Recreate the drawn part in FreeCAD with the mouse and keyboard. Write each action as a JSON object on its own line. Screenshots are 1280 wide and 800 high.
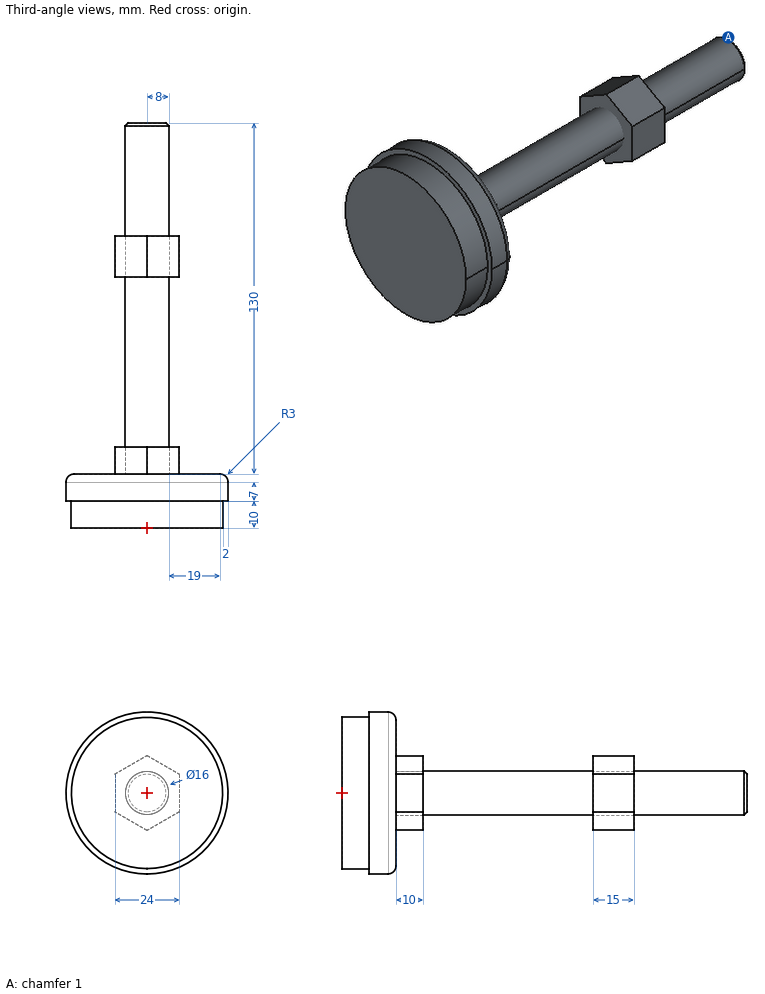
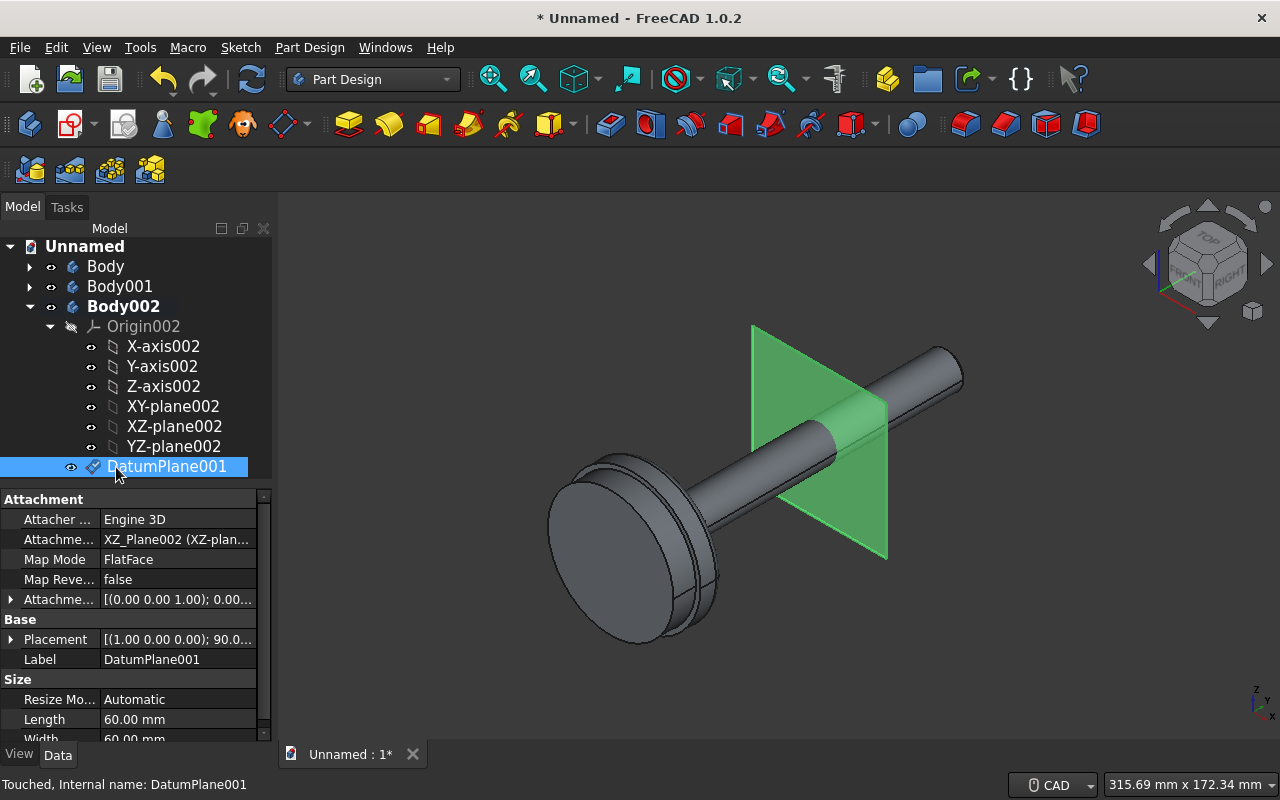
{"action": "left_click", "coordinate": [70, 124]}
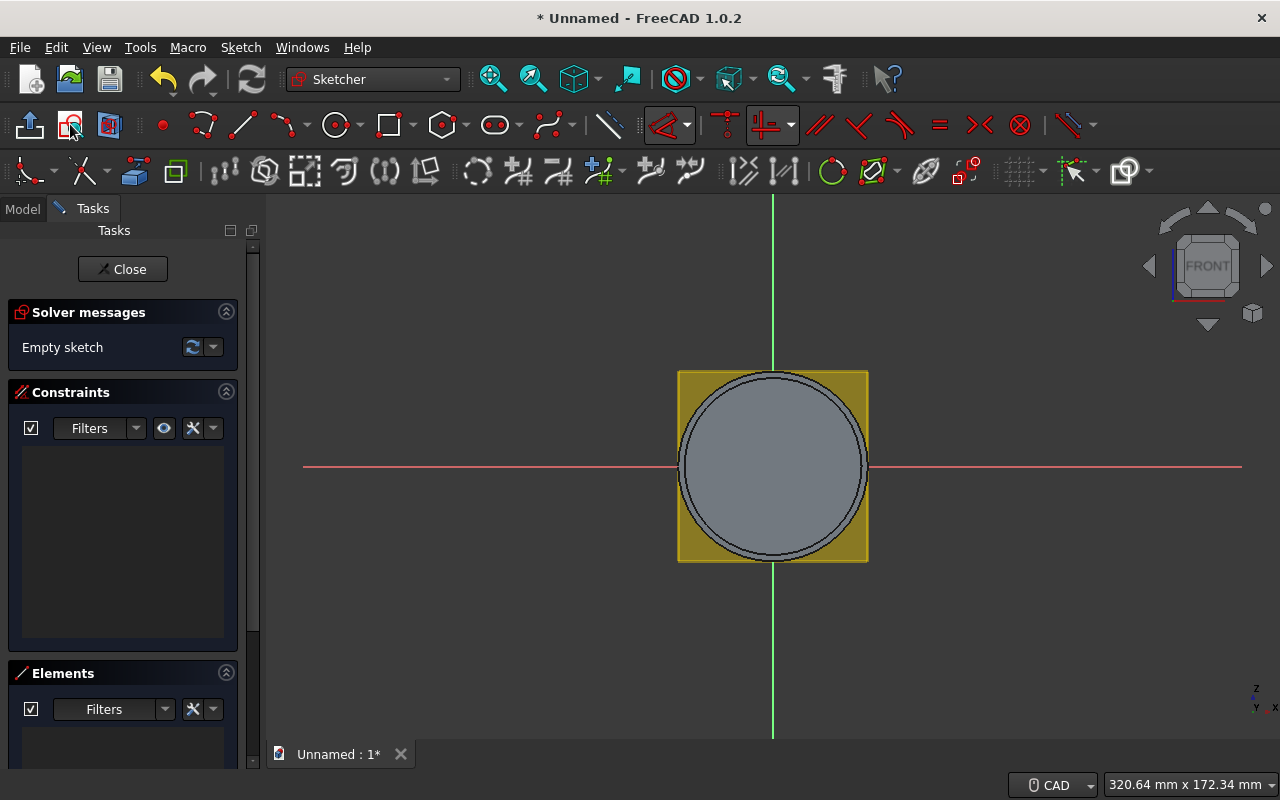
{"action": "scroll", "coordinate": [795, 467], "scroll_direction": "up", "scroll_amount": 7}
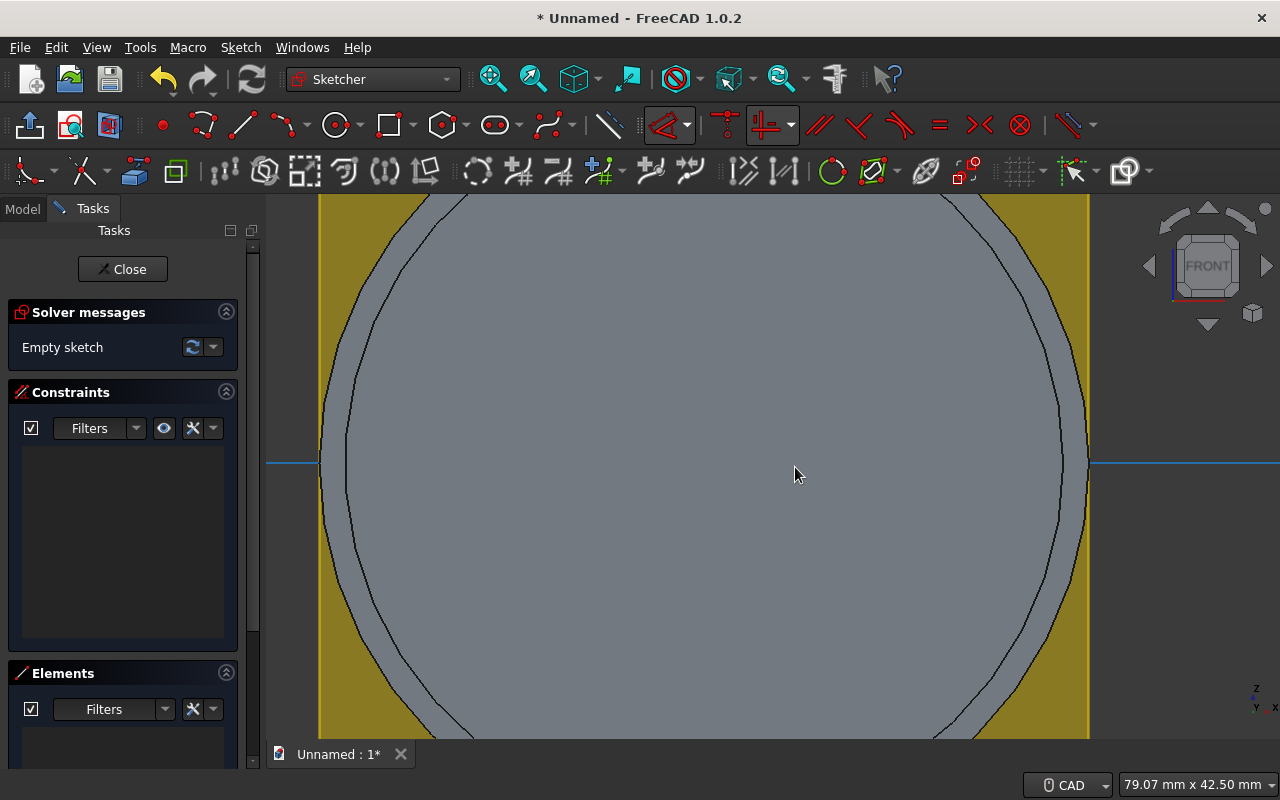
{"action": "left_click", "coordinate": [442, 126]}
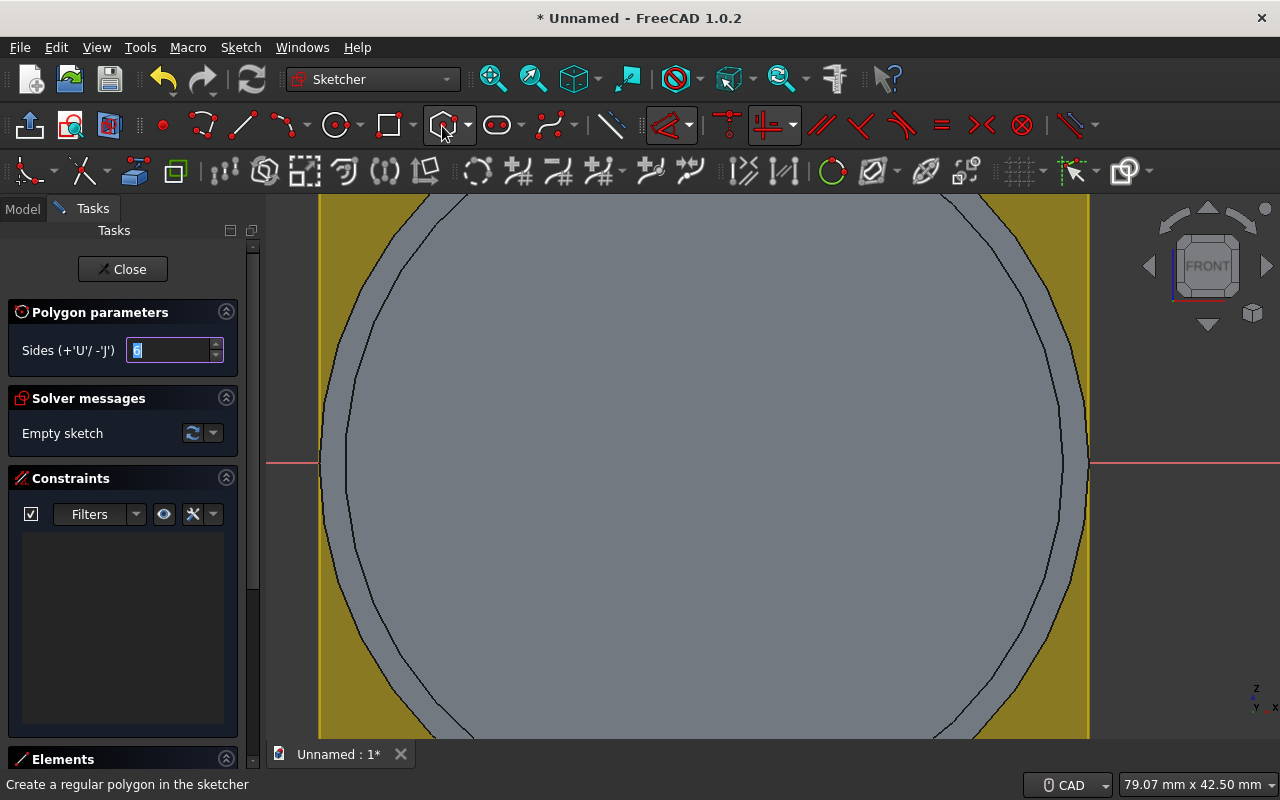
{"action": "left_click", "coordinate": [704, 463]}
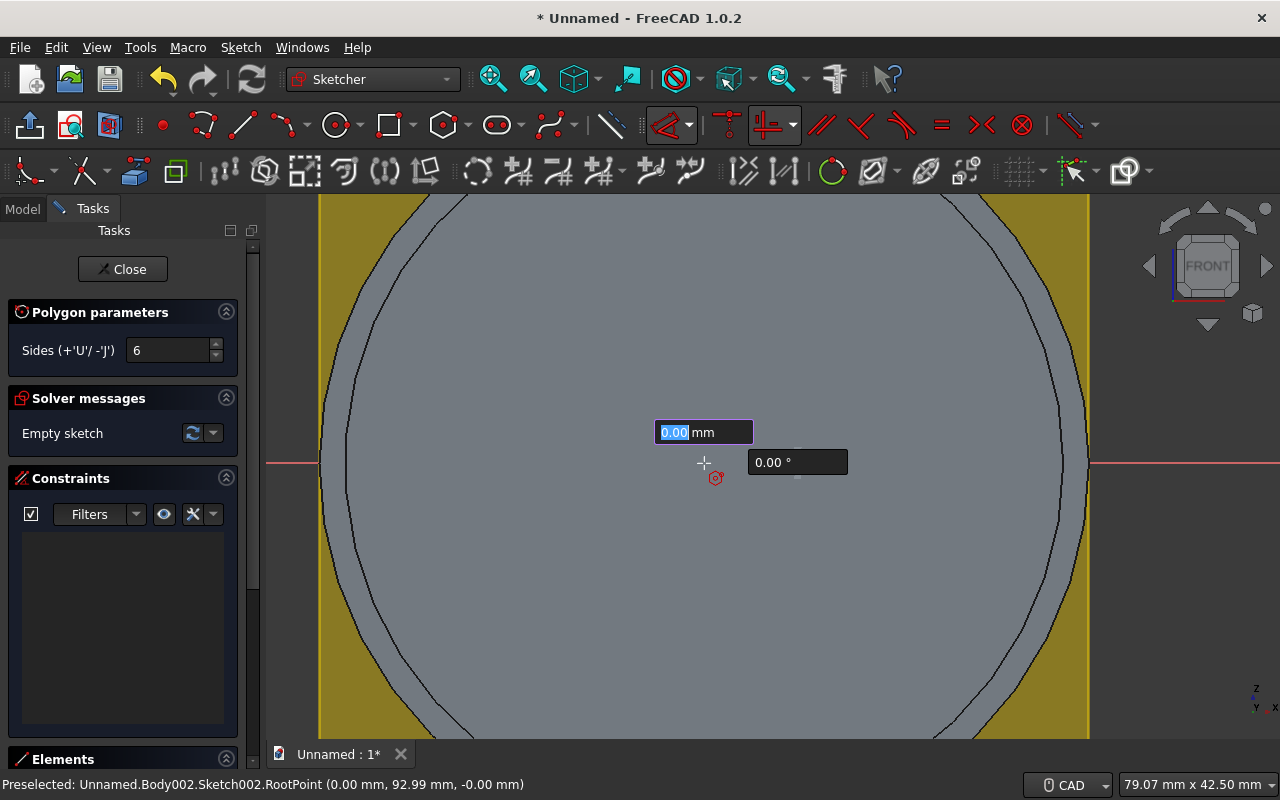
{"action": "left_click", "coordinate": [704, 641]}
{"action": "key", "text": "Escape"}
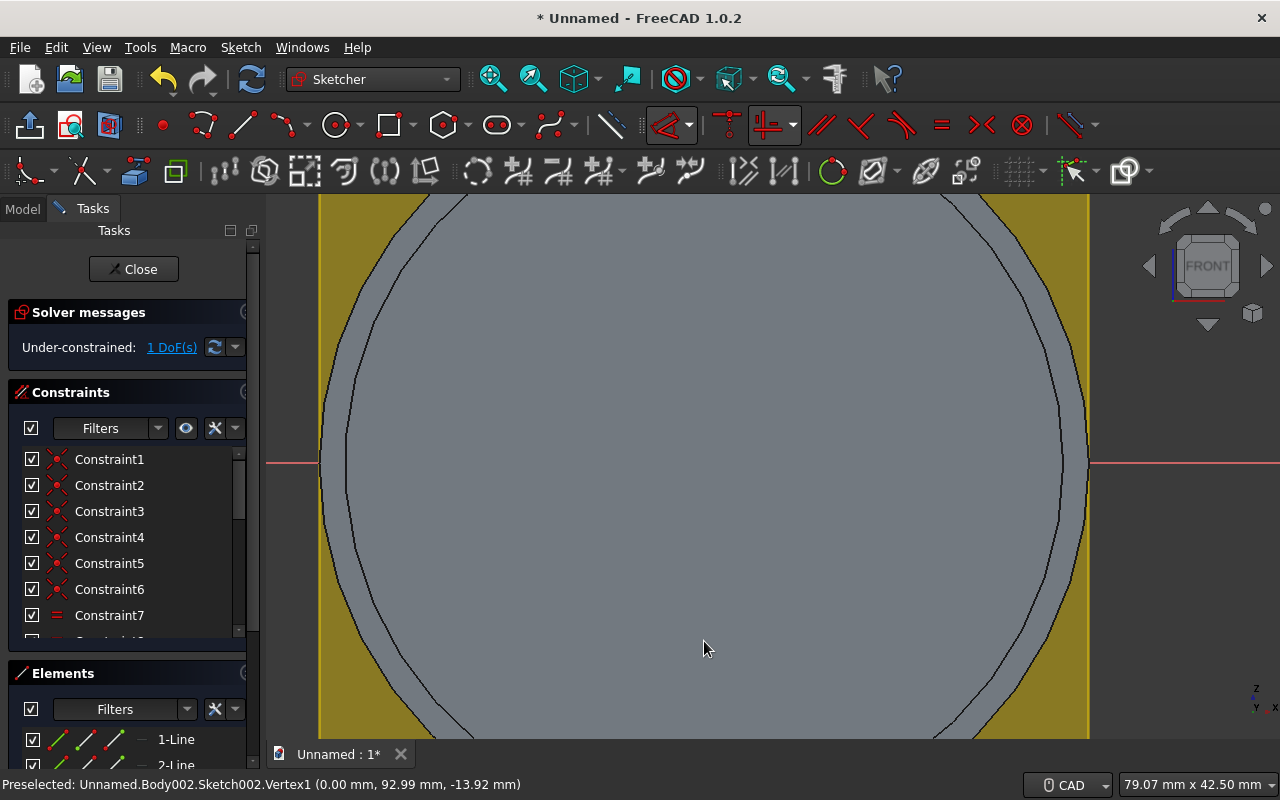
{"action": "left_click", "coordinate": [550, 374]}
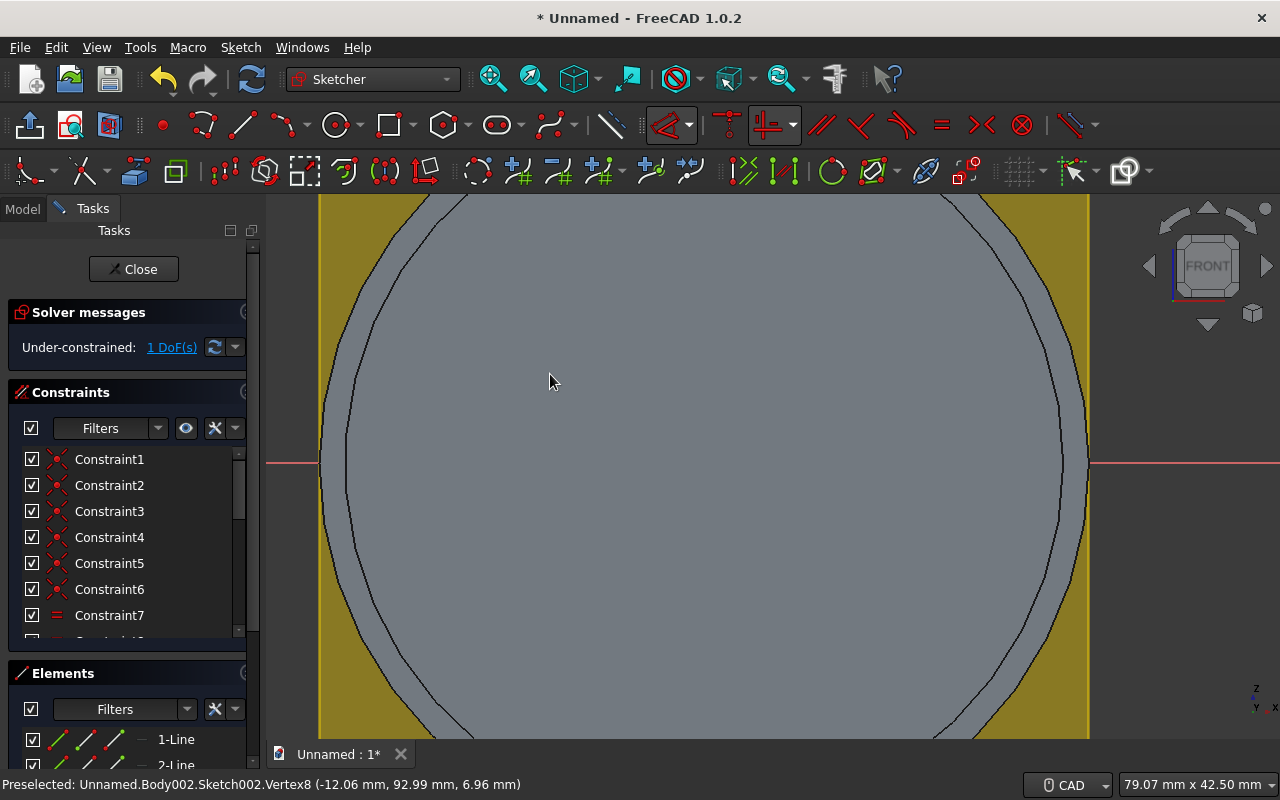
{"action": "left_click", "coordinate": [859, 553]}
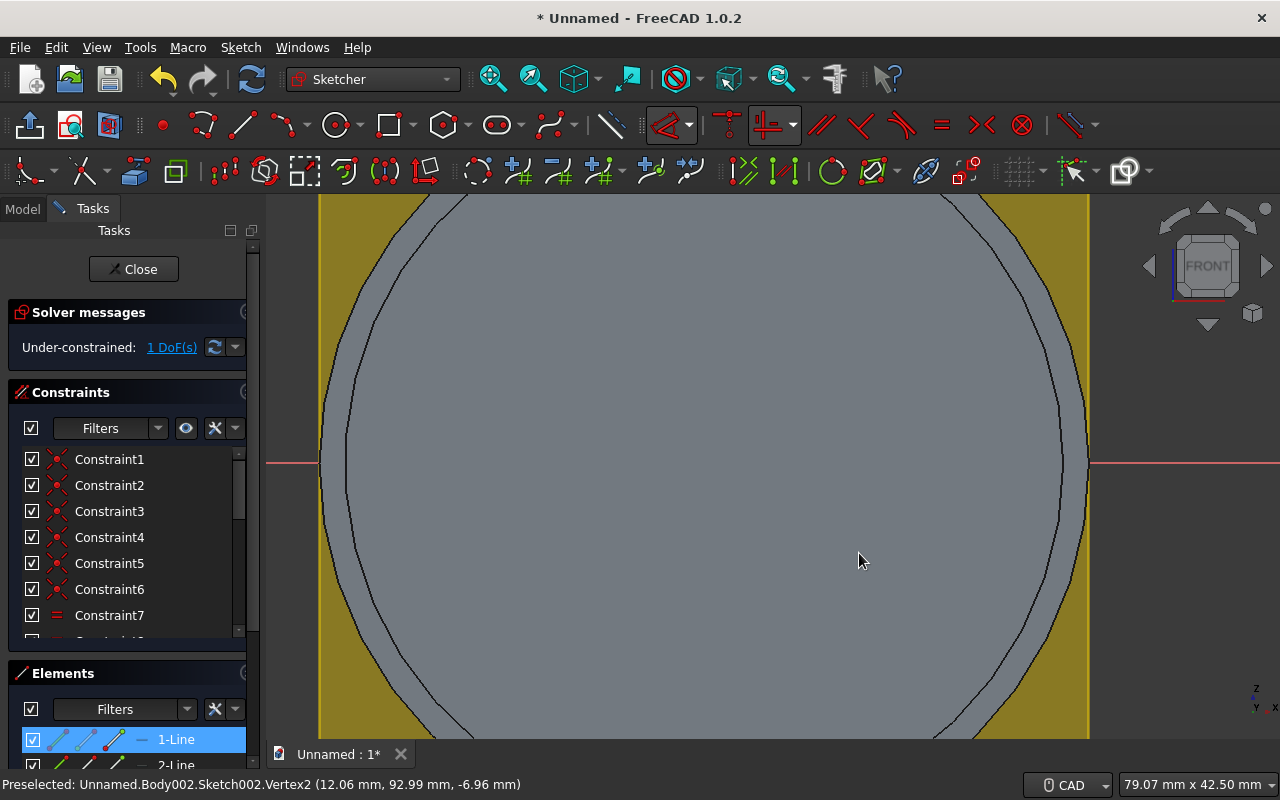
{"action": "key", "text": "l"}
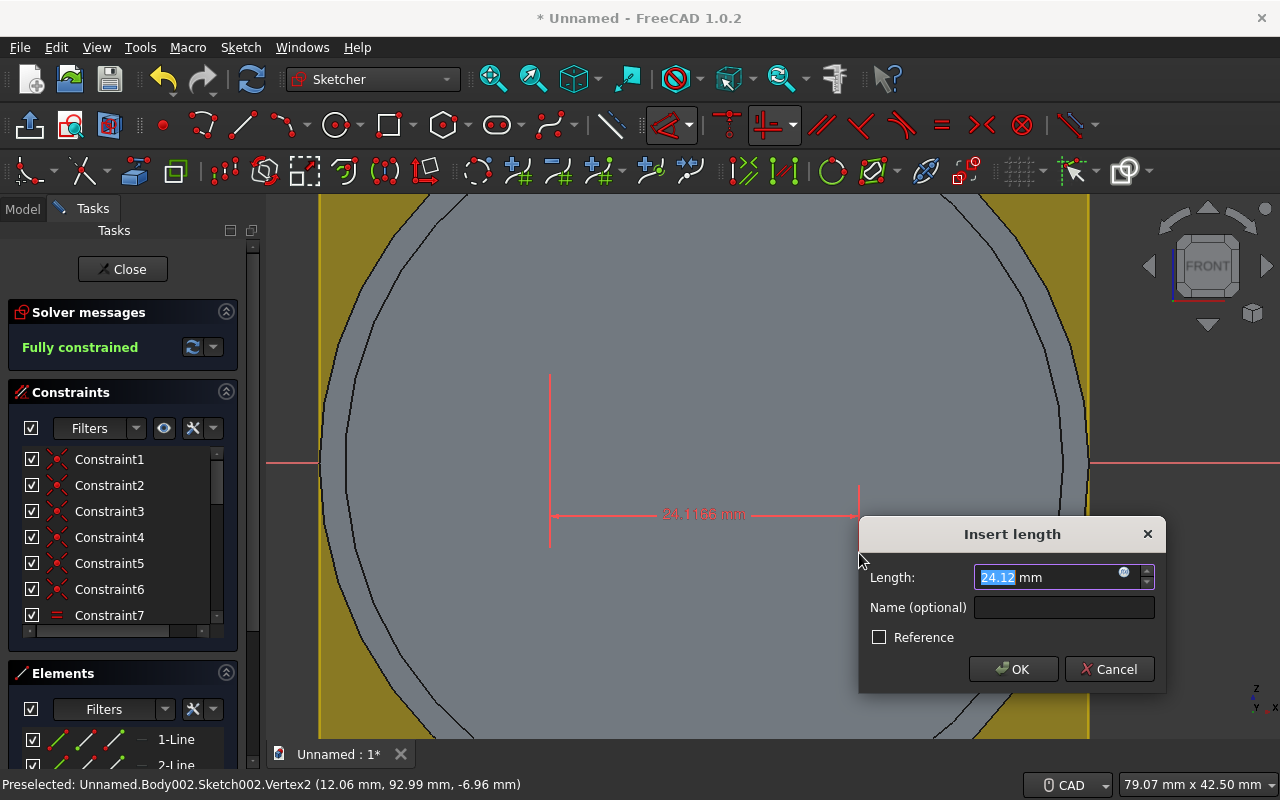
{"action": "type", "text": "24"}
{"action": "key", "text": "Return"}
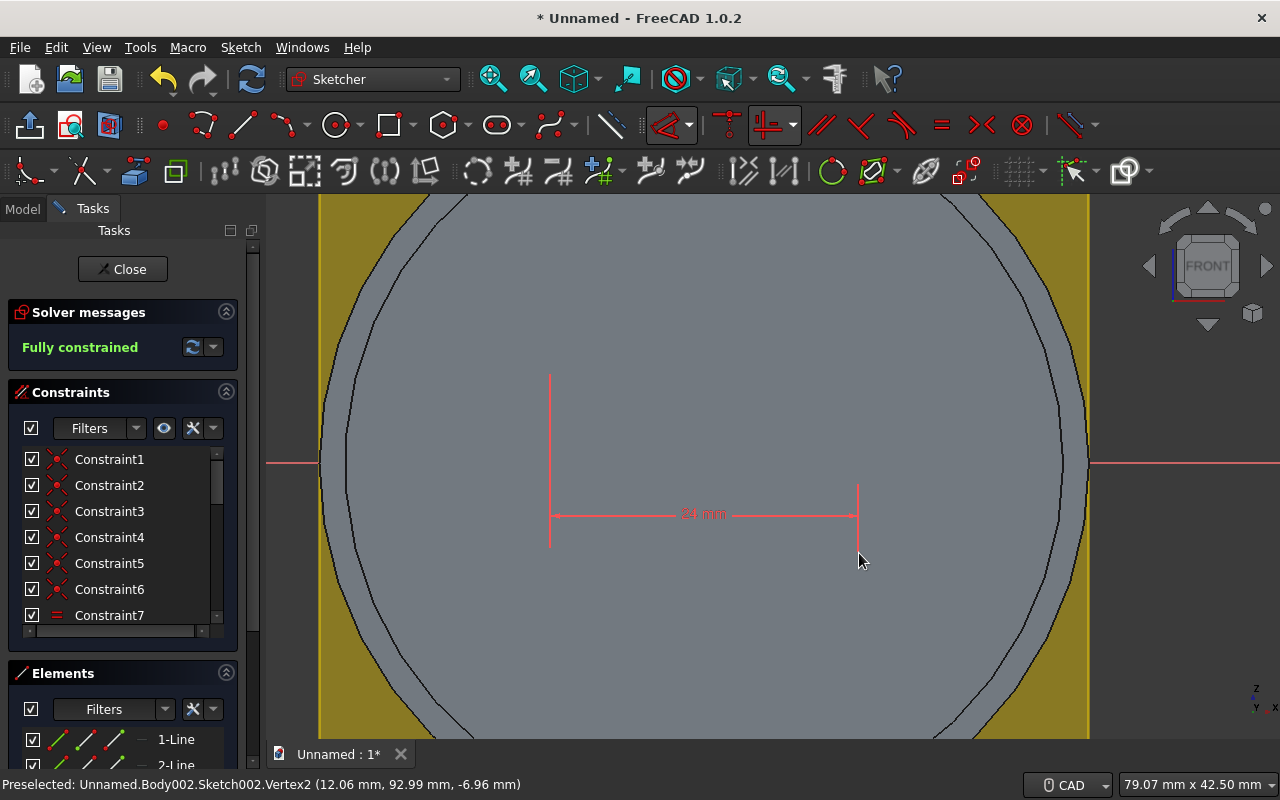
{"action": "left_click", "coordinate": [123, 269]}